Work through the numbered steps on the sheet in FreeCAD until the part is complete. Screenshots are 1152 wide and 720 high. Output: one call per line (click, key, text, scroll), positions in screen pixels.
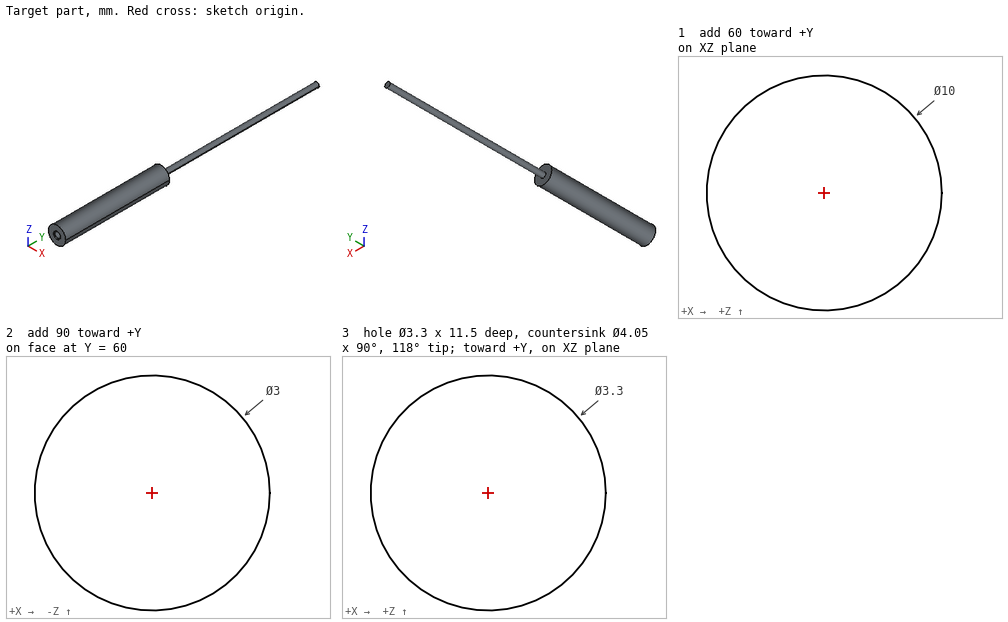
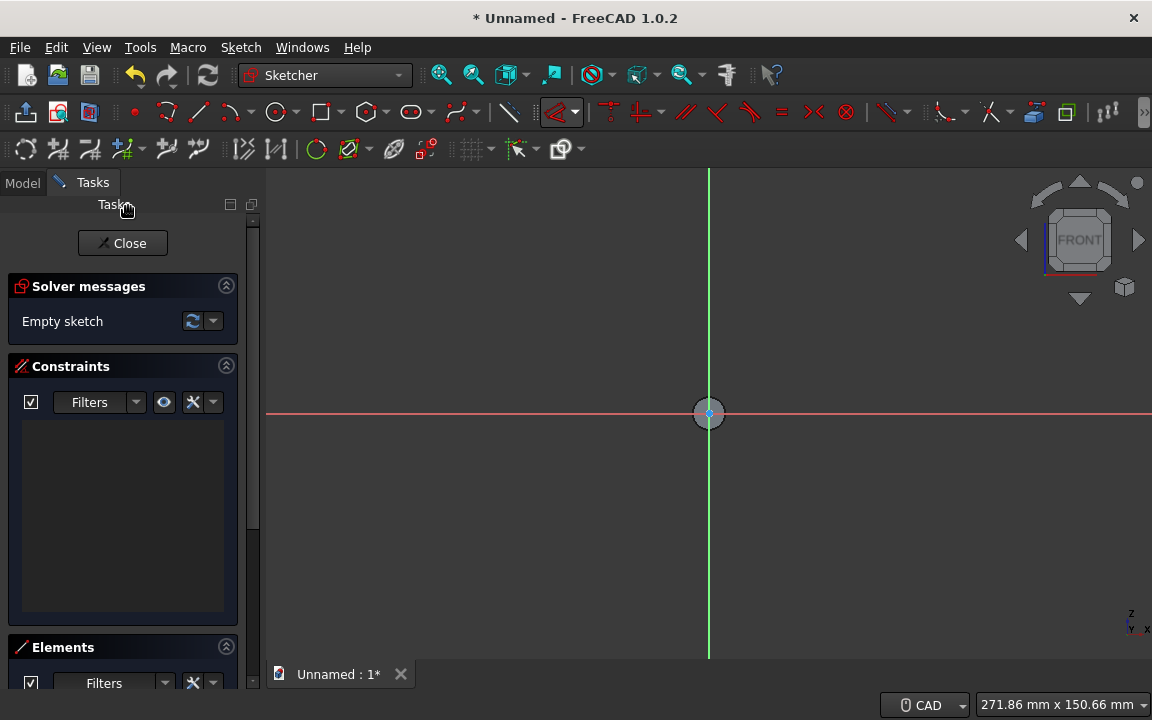
scroll(713, 414, up, 15)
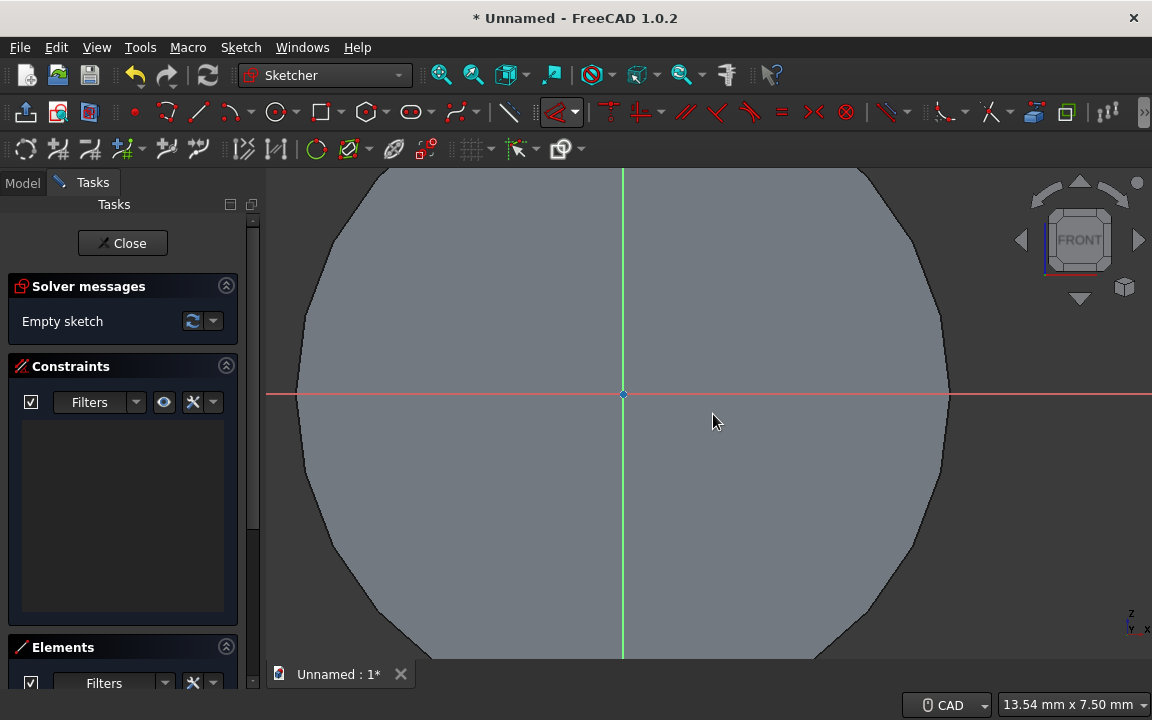
scroll(587, 355, up, 2)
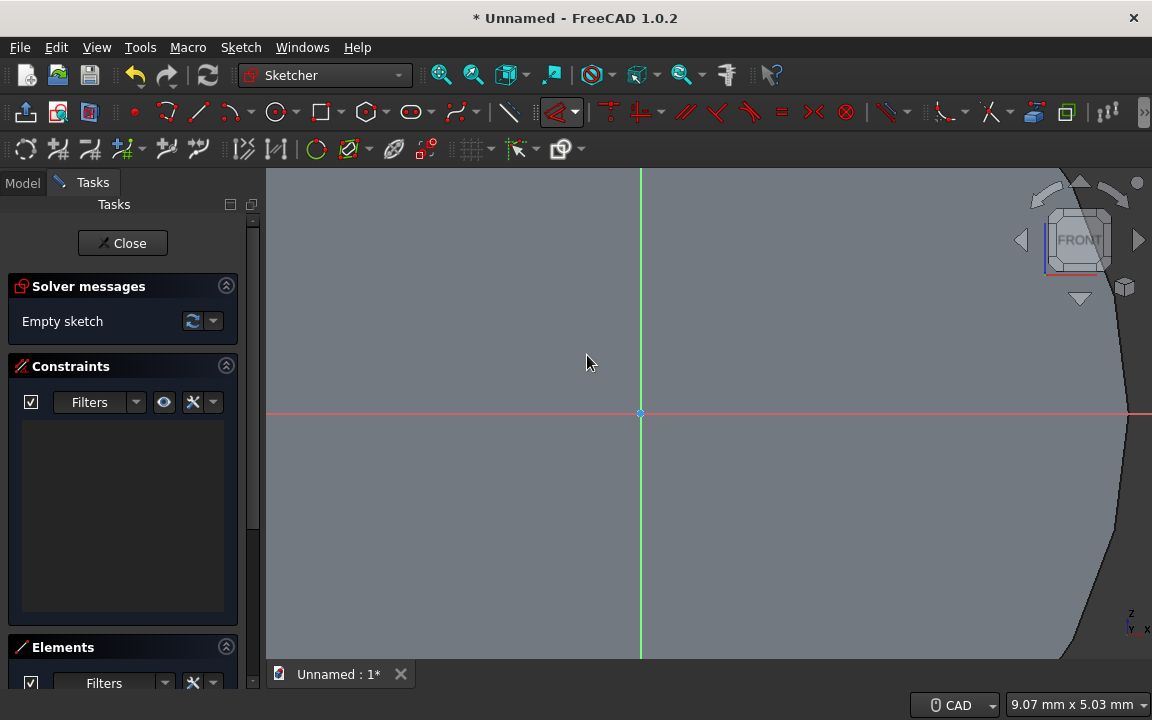
click(276, 112)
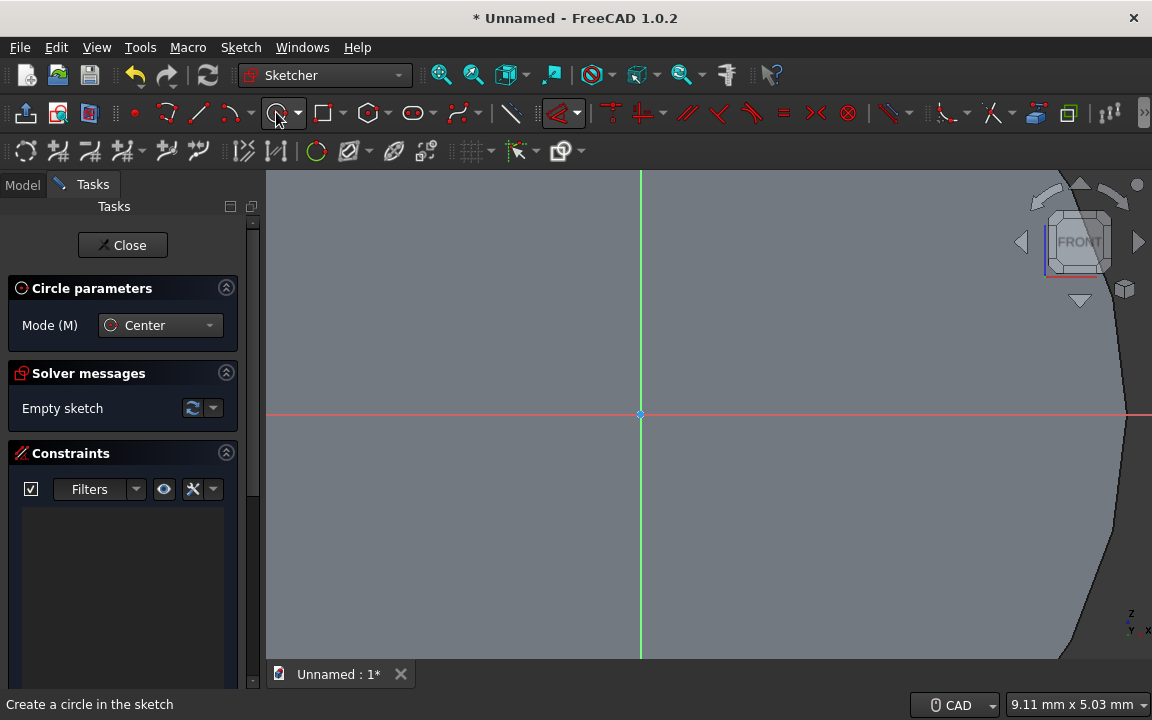
click(641, 415)
click(754, 301)
key(Escape)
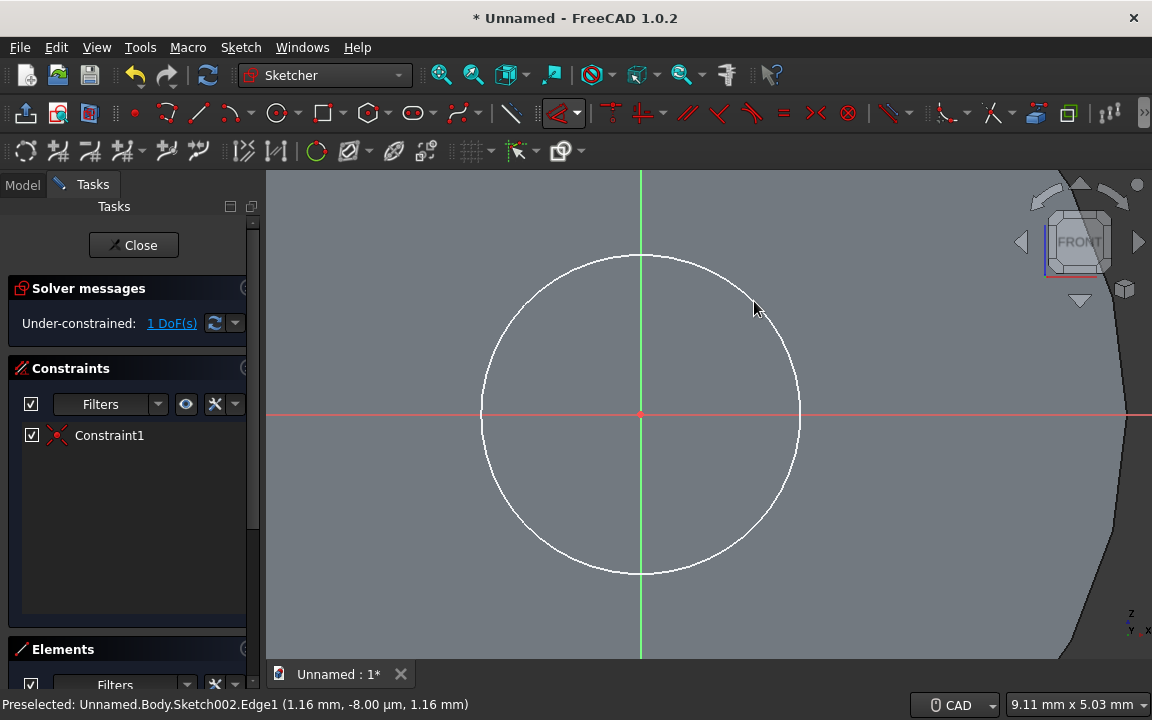
click(753, 301)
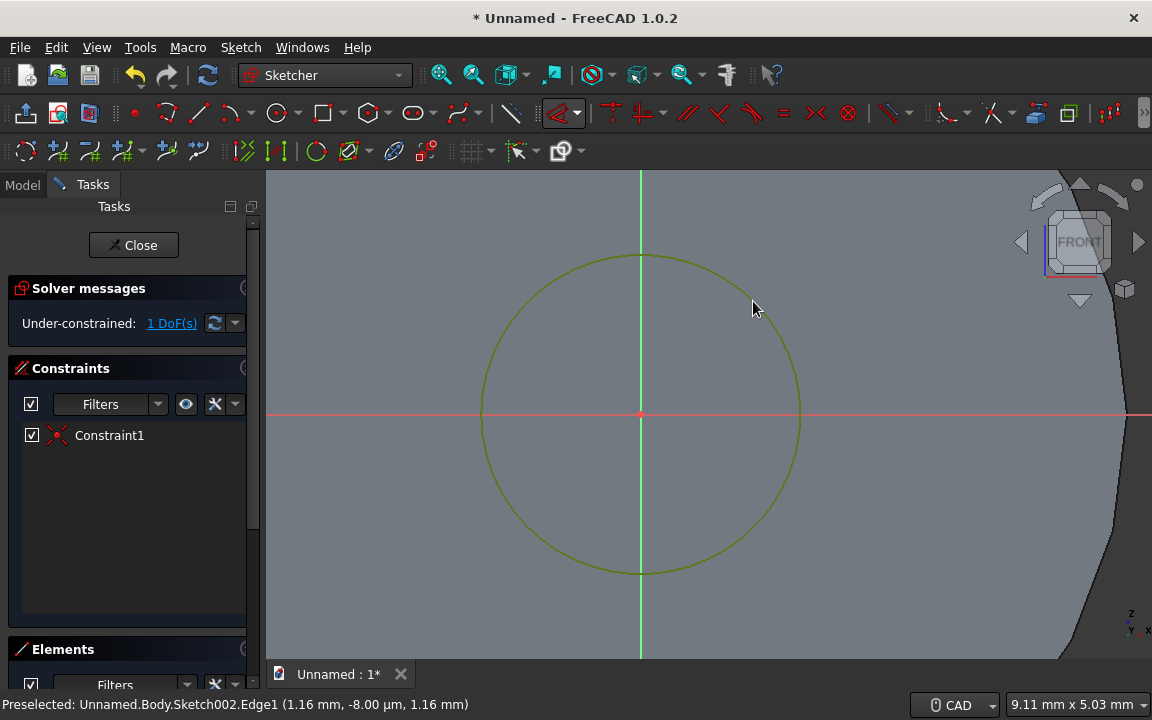
click(580, 114)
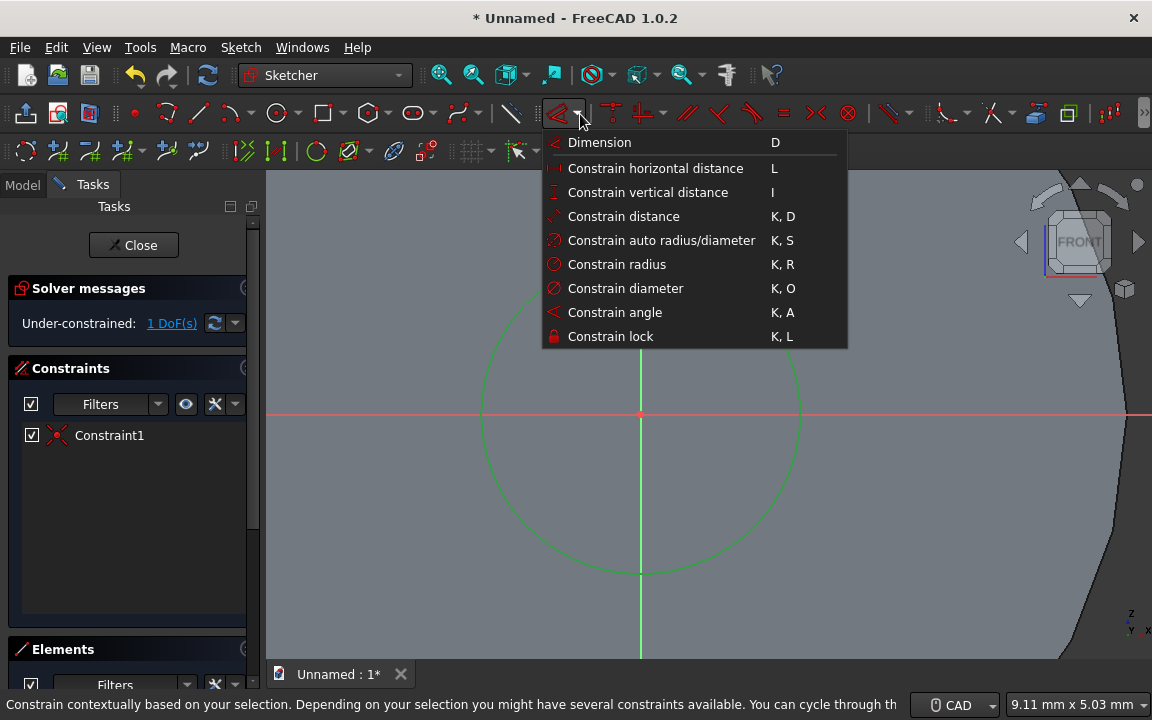
click(695, 288)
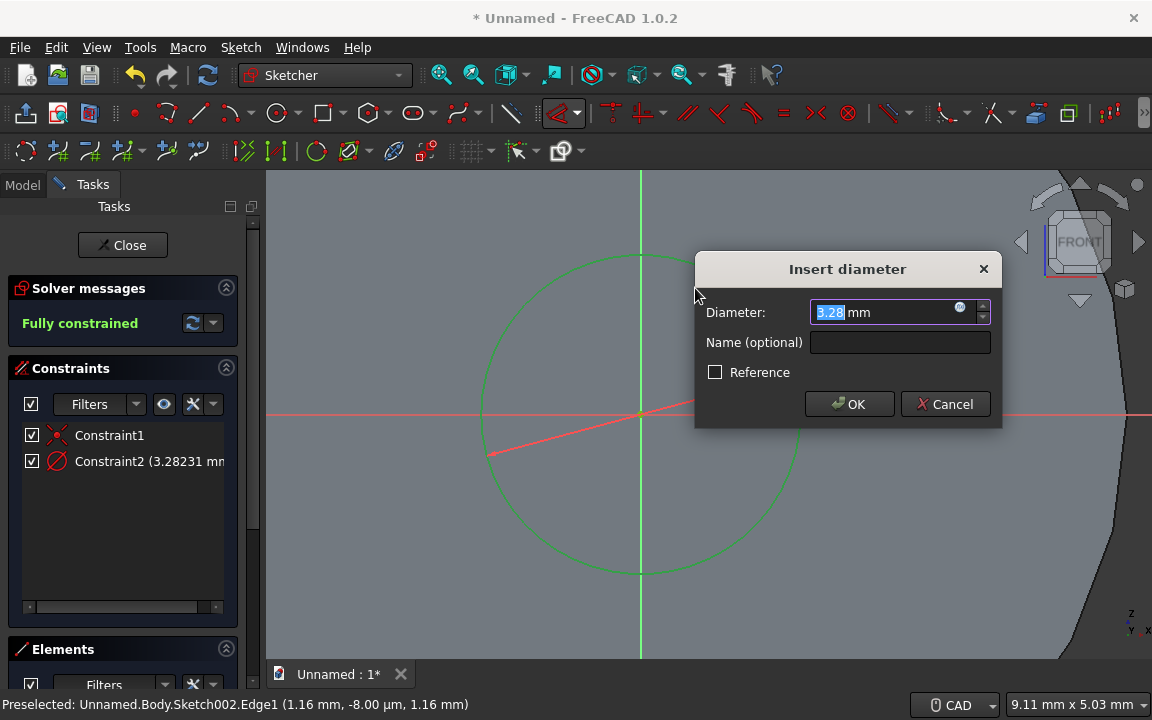
text(3.3)
key(Return)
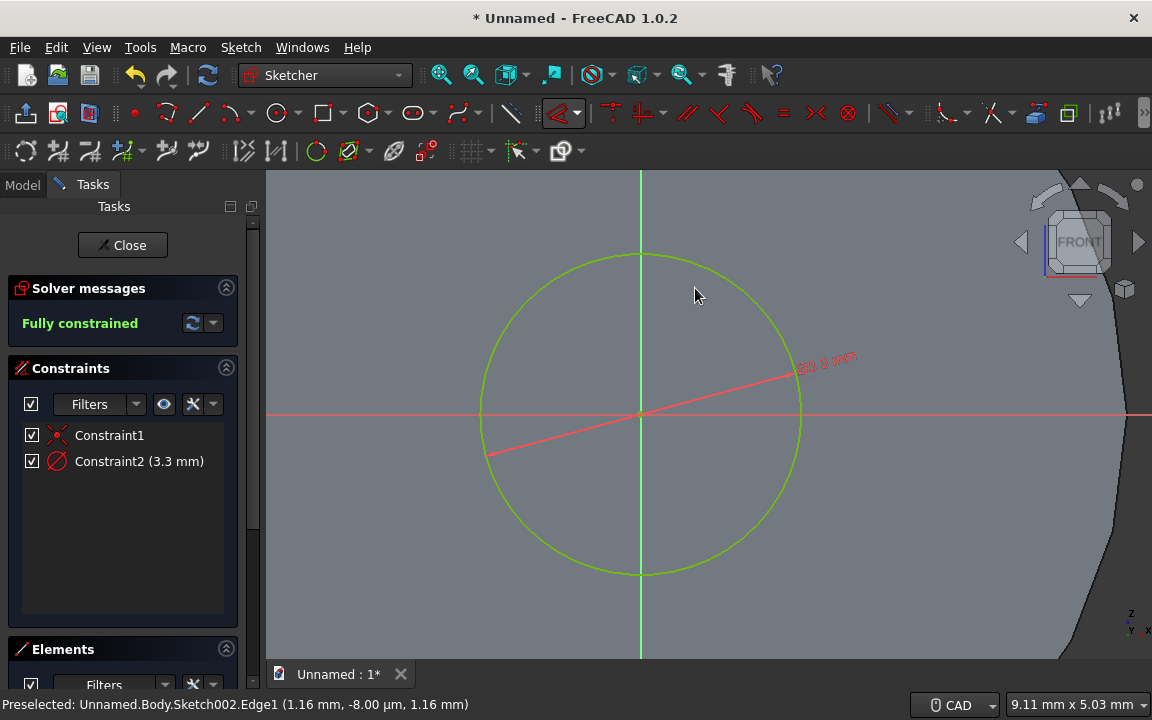
click(123, 245)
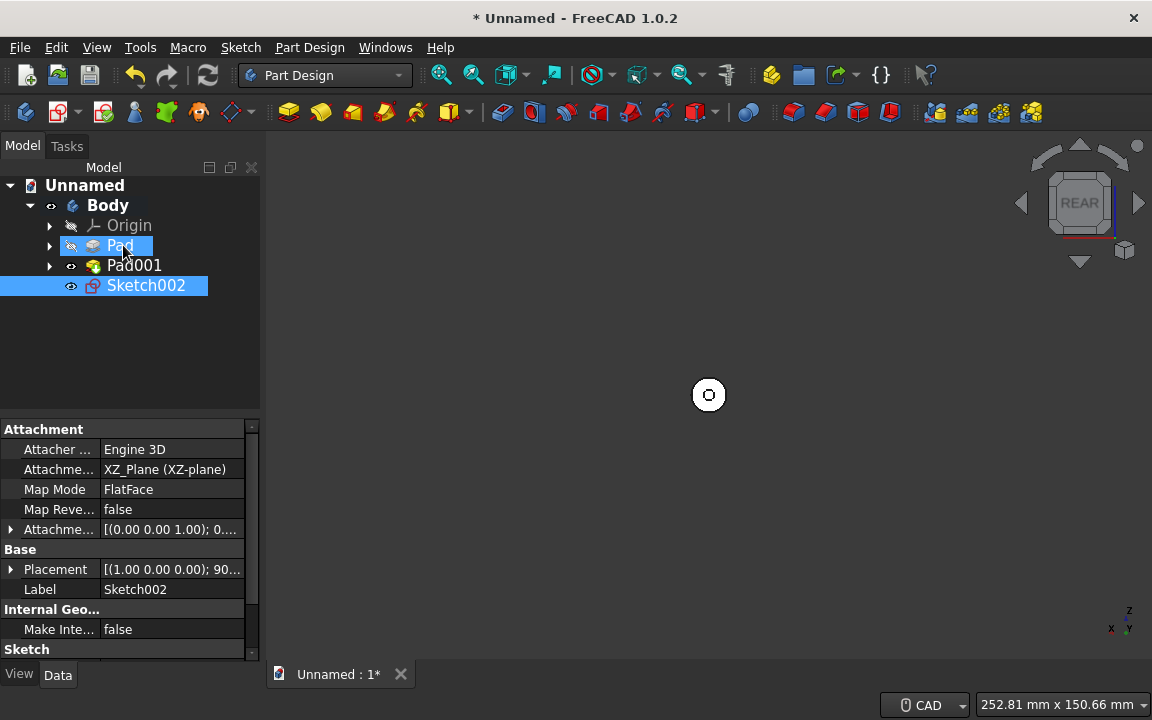
click(536, 112)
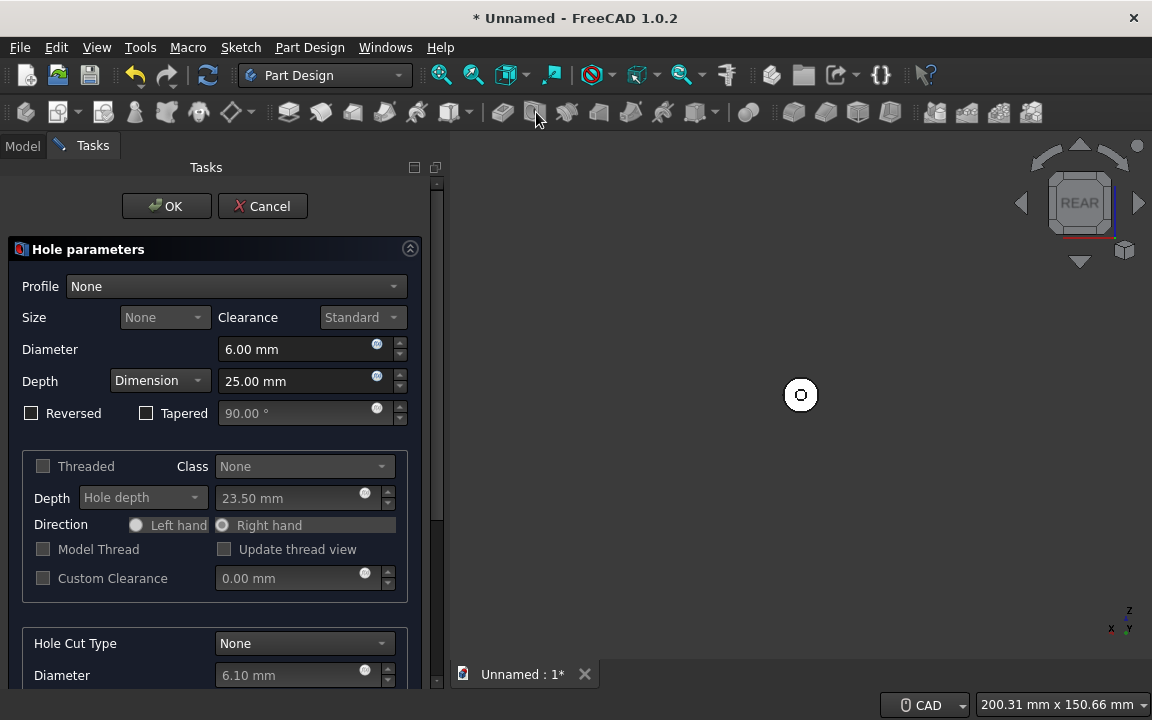
triple_click(305, 349)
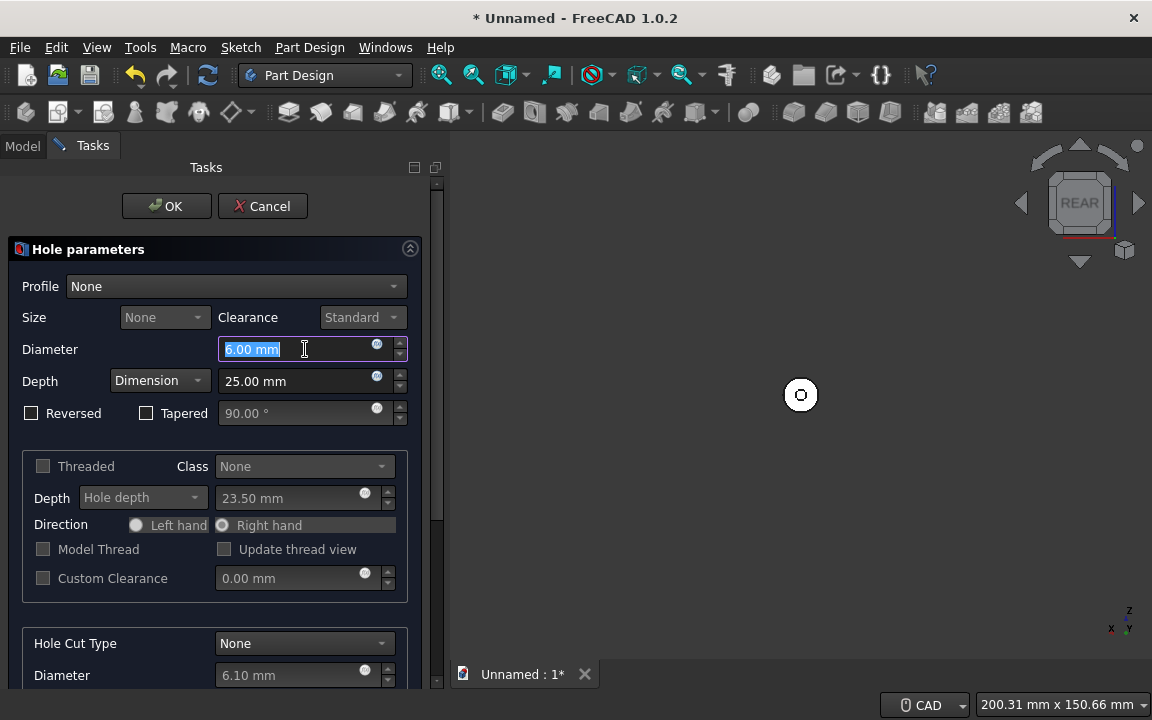
text(3.3)
key(Tab)